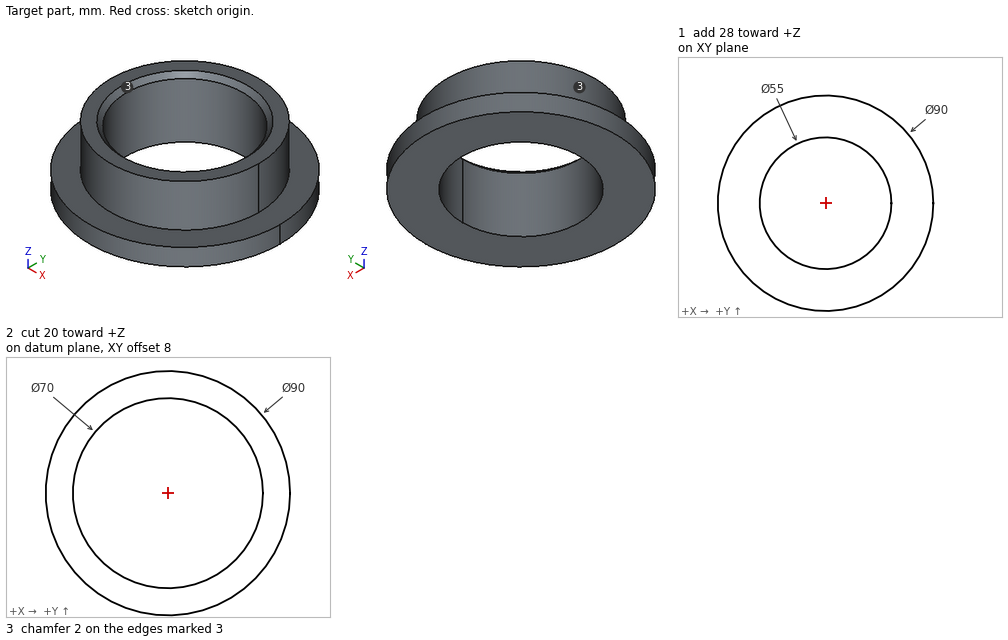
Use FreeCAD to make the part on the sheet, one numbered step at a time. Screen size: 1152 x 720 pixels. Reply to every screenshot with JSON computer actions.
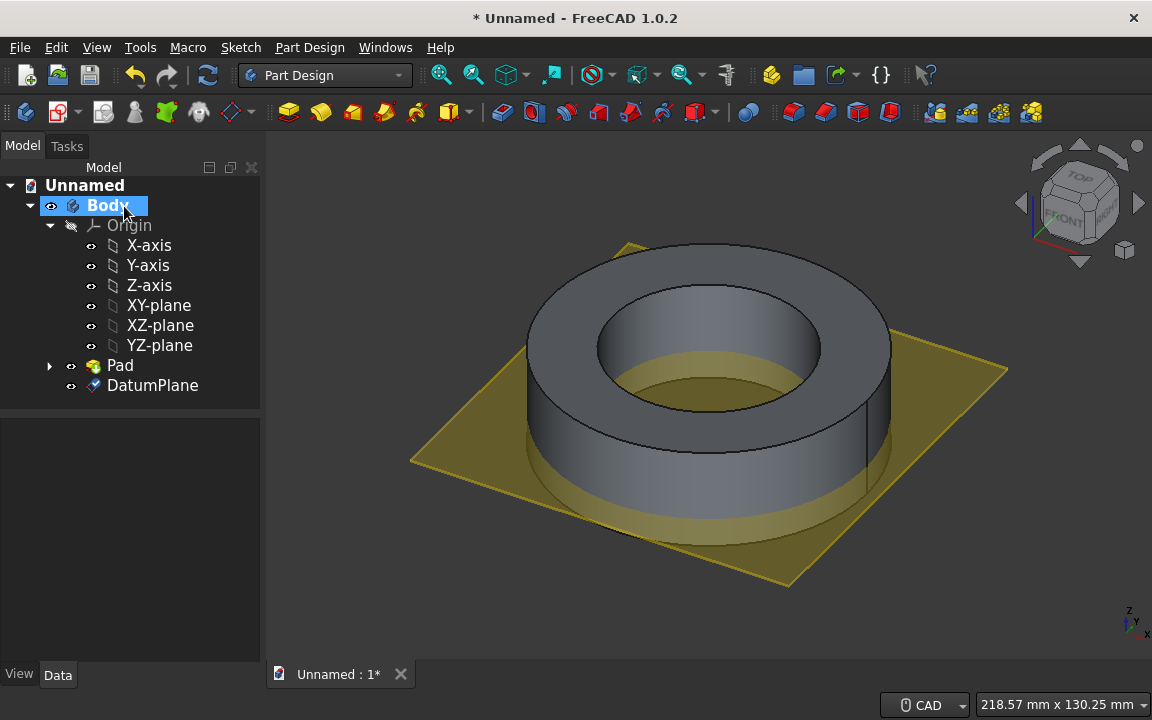
{"action": "left_click", "coordinate": [116, 386]}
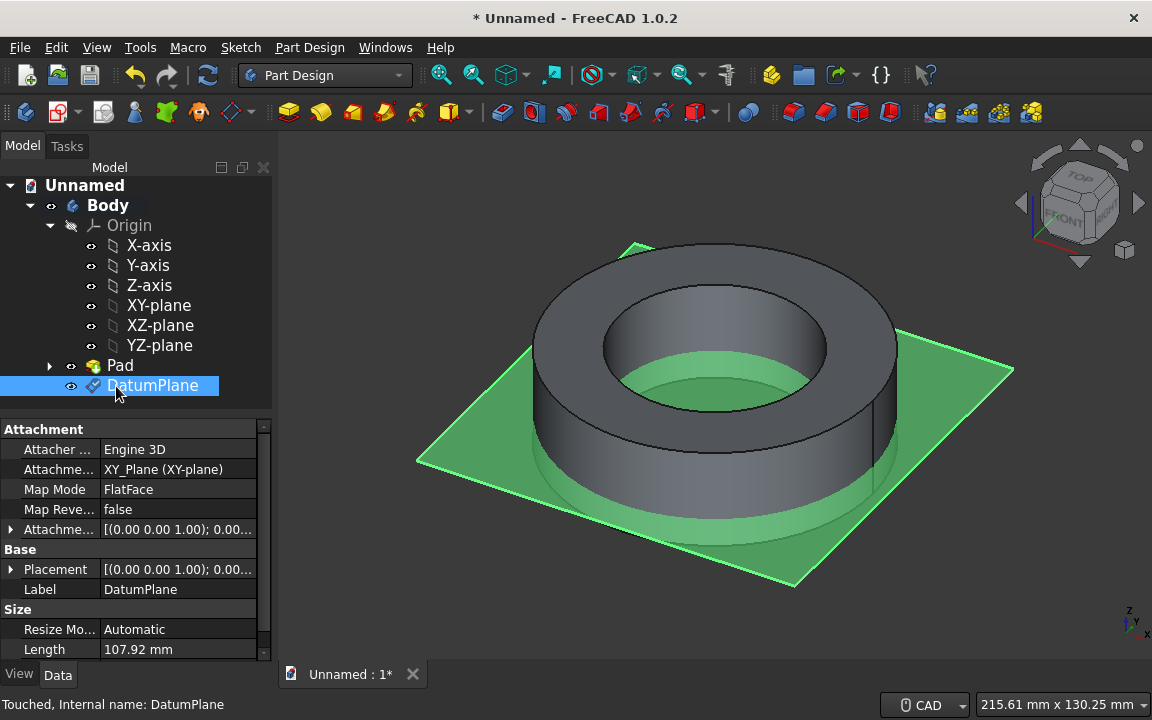
{"action": "left_click", "coordinate": [58, 112]}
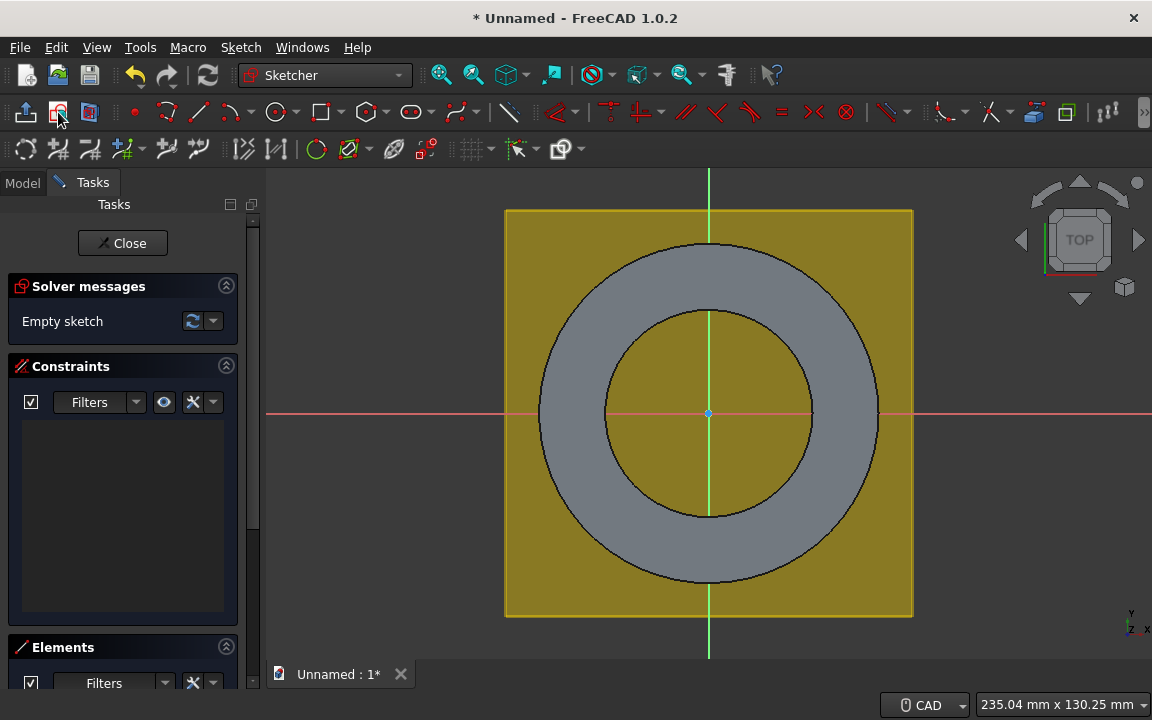
{"action": "left_click", "coordinate": [90, 112]}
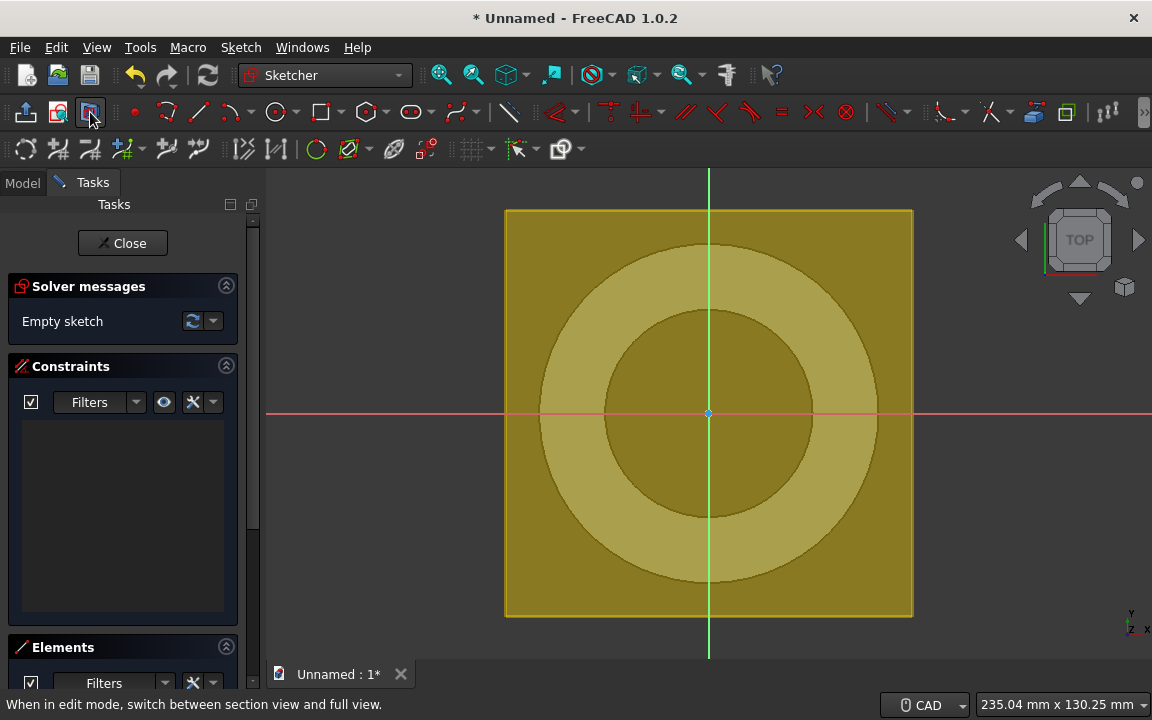
{"action": "left_click", "coordinate": [276, 112]}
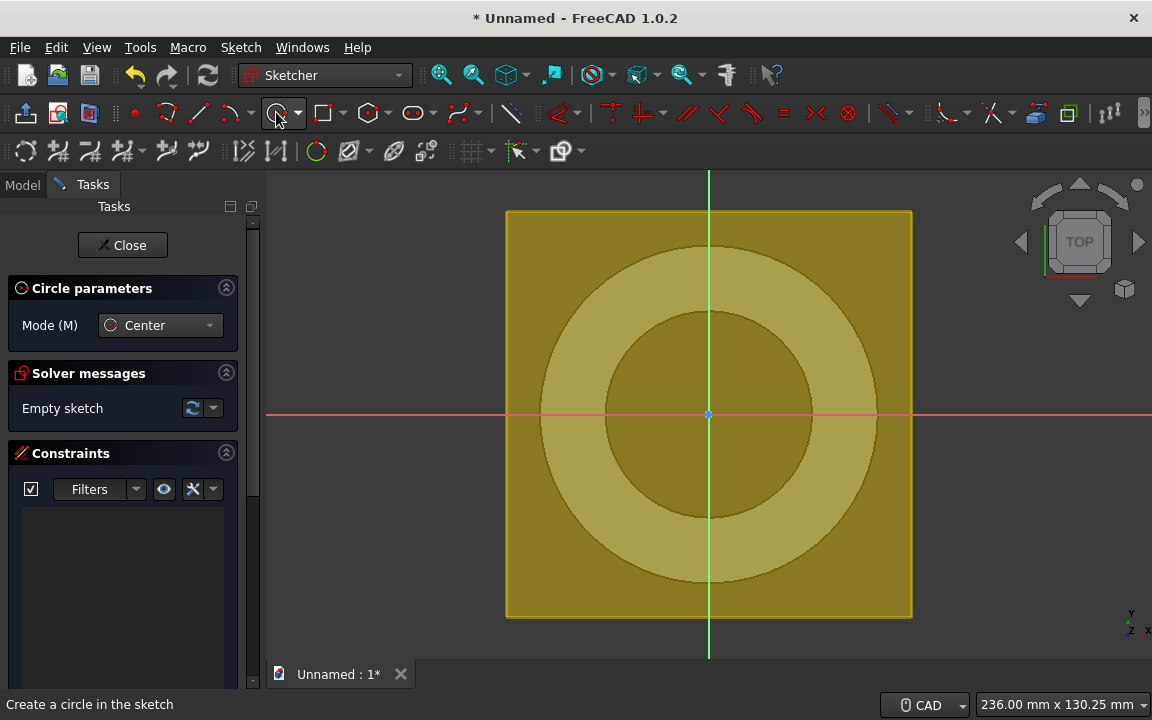
{"action": "left_click", "coordinate": [709, 414]}
{"action": "mouse_move", "coordinate": [828, 295]}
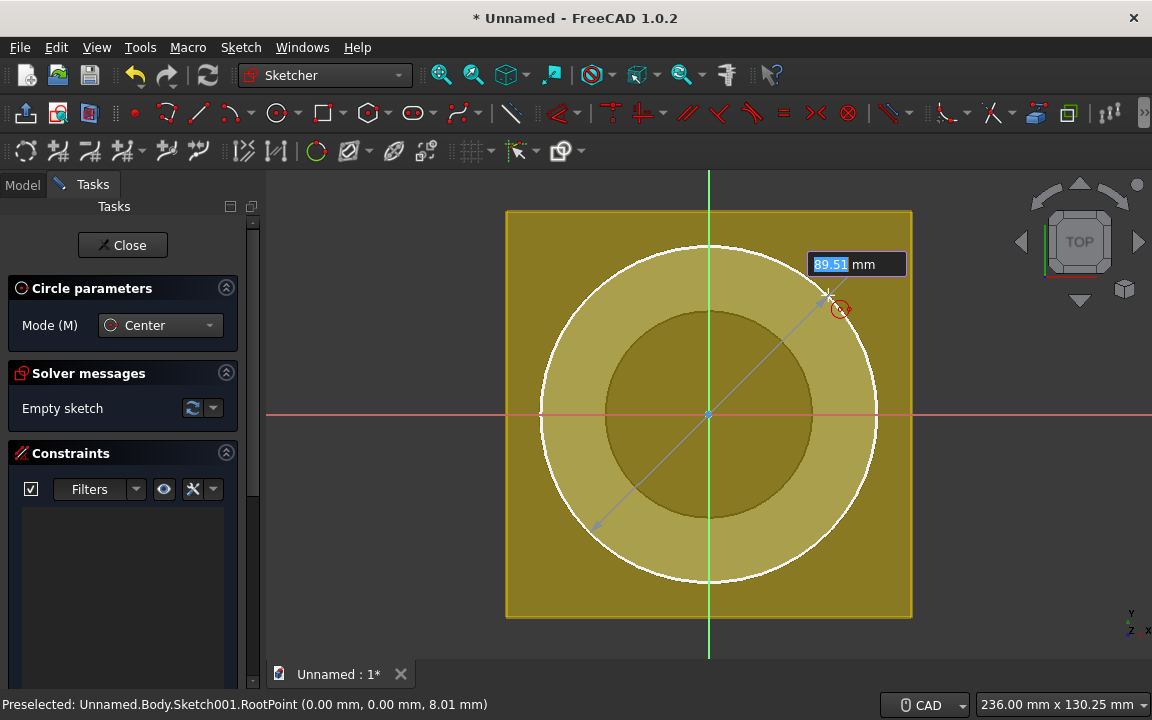
{"action": "type", "text": "90"}
{"action": "key", "text": "Return"}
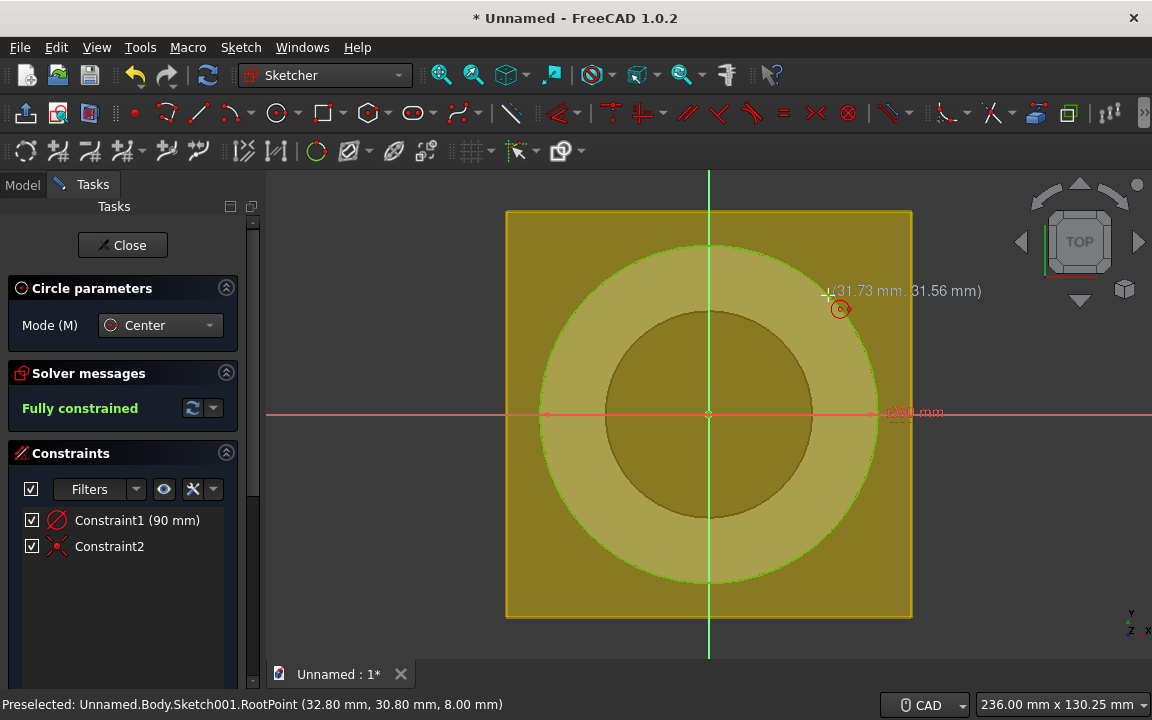
{"action": "left_click", "coordinate": [709, 414]}
{"action": "mouse_move", "coordinate": [802, 322]}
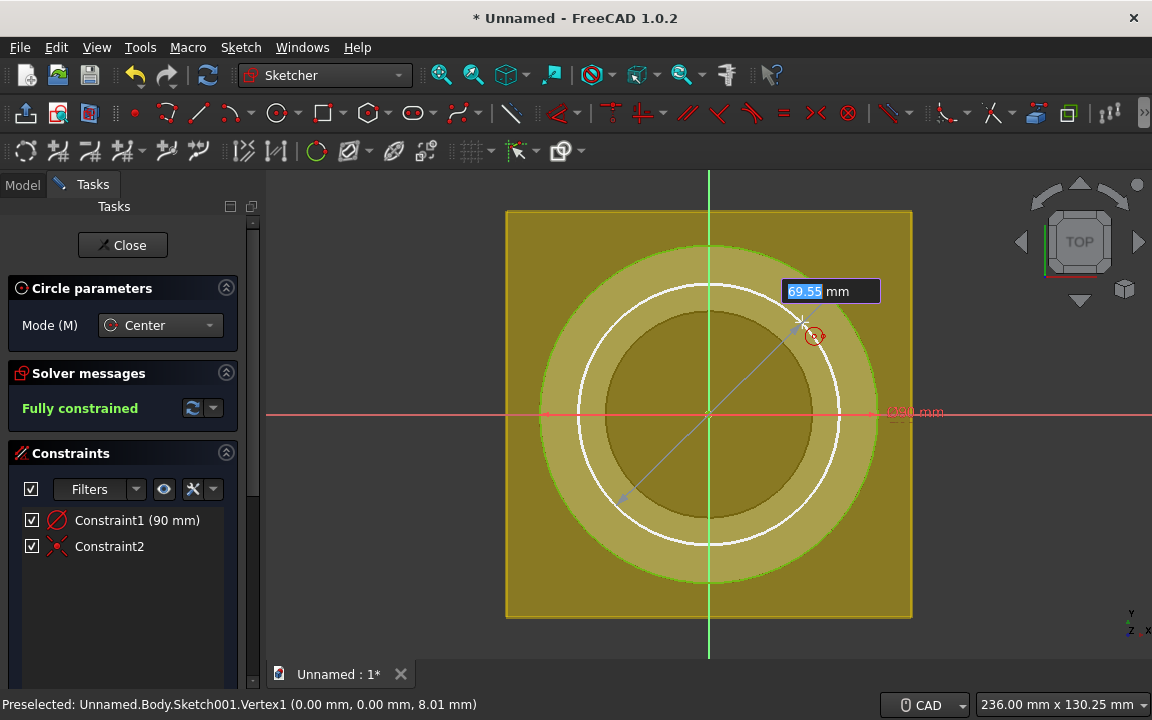
{"action": "type", "text": "70"}
{"action": "key", "text": "Return"}
{"action": "key", "text": "Escape"}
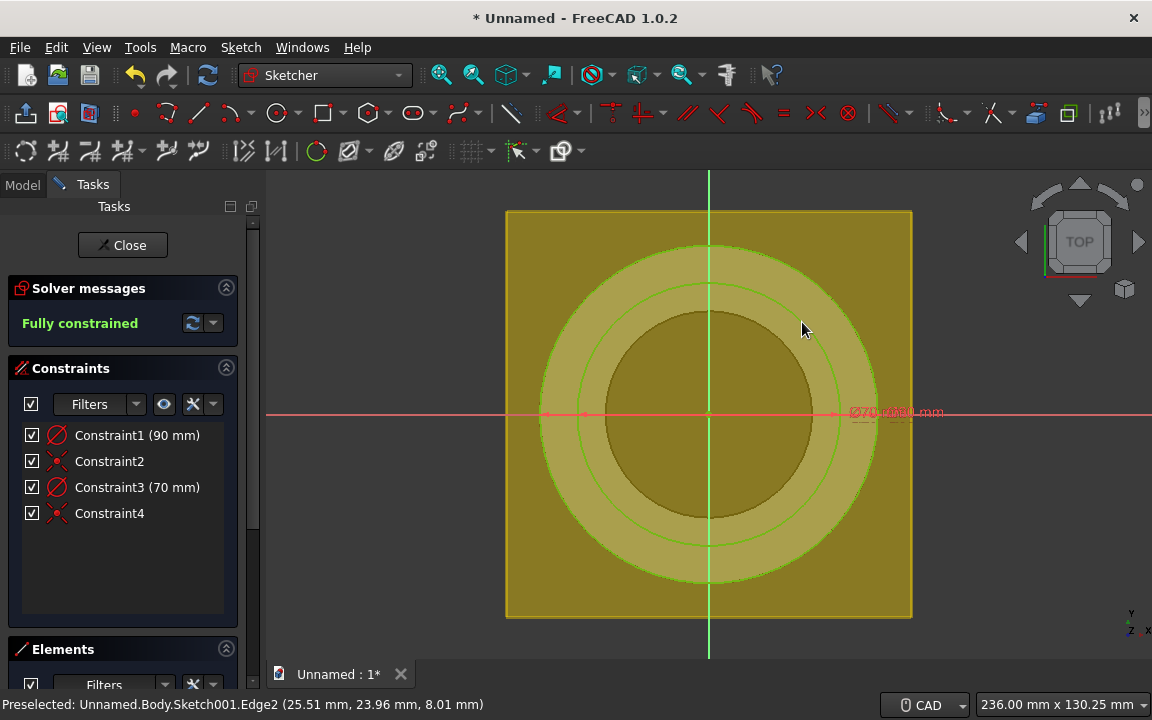
{"action": "left_click", "coordinate": [123, 245]}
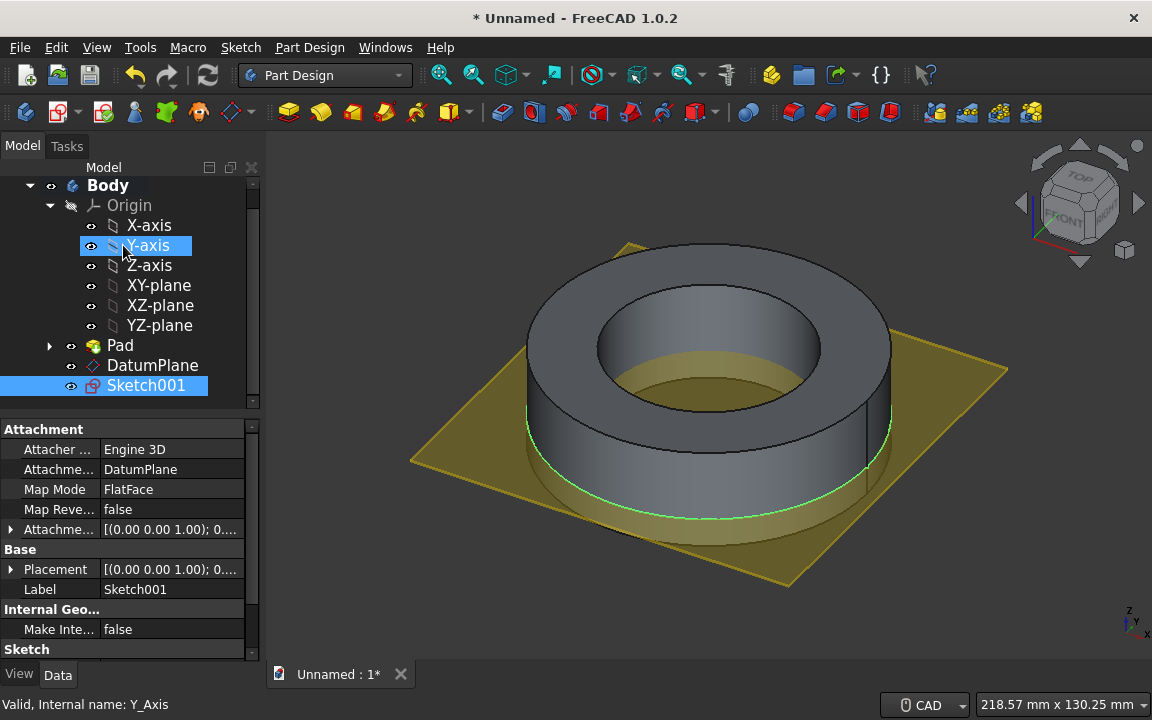
{"action": "left_click", "coordinate": [504, 112]}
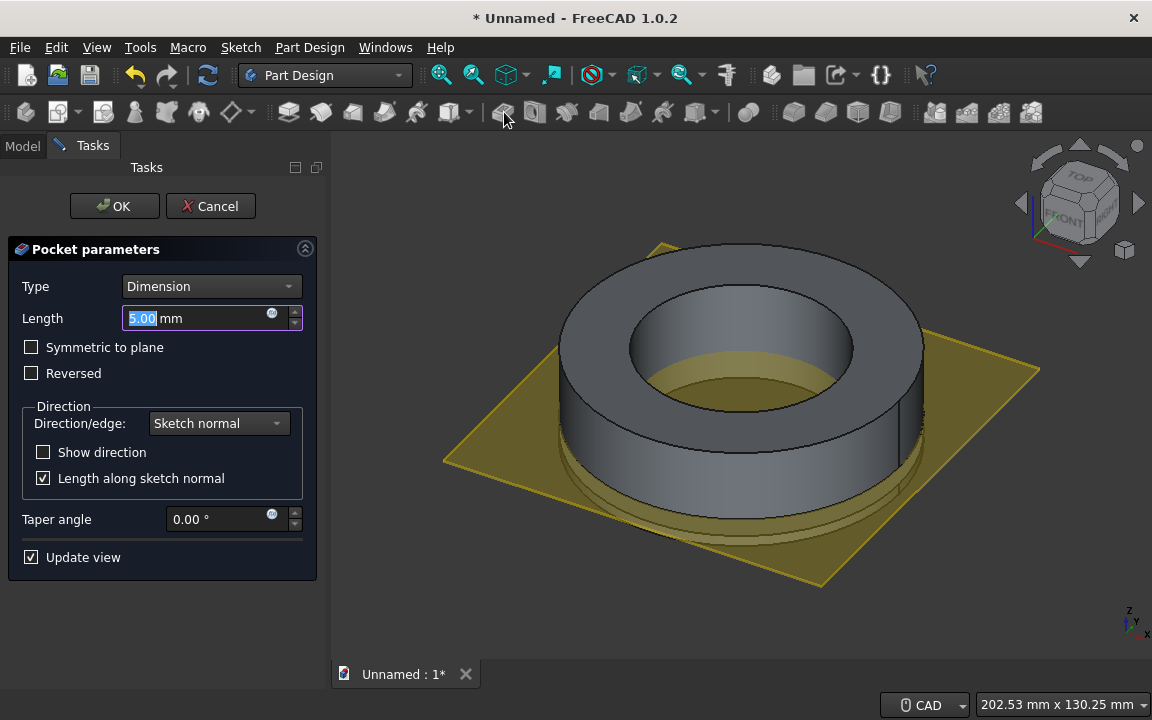
{"action": "type", "text": "20"}
{"action": "key", "text": "Tab"}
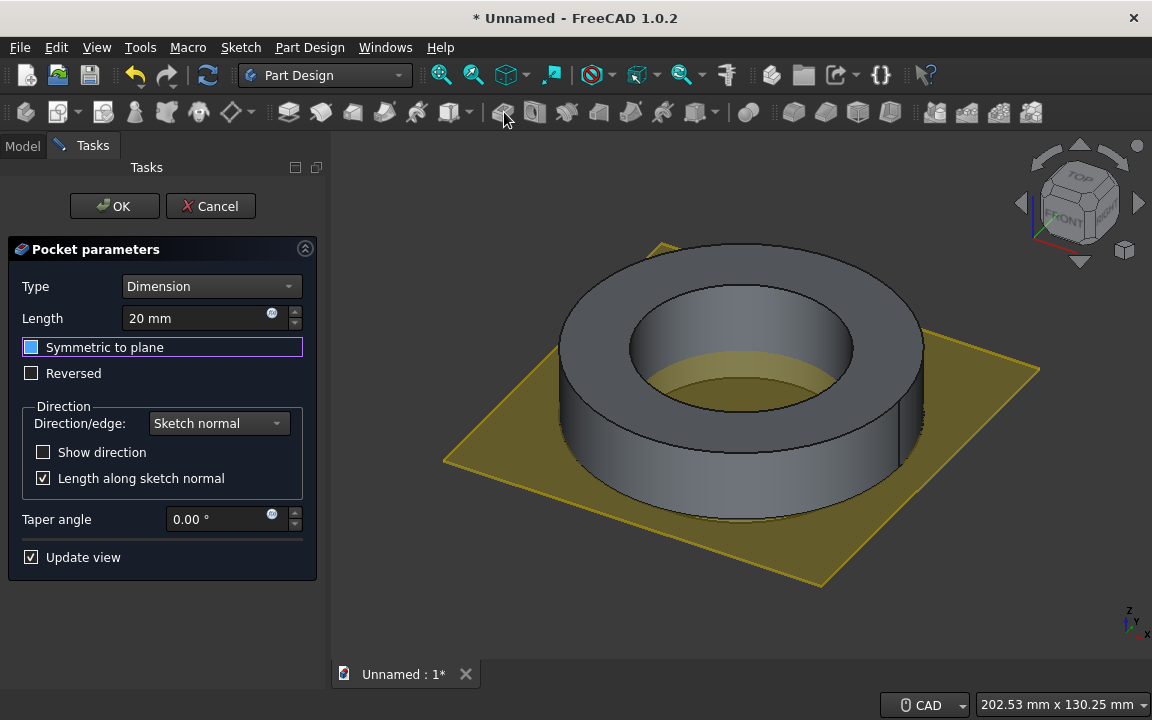
{"action": "left_click", "coordinate": [30, 373]}